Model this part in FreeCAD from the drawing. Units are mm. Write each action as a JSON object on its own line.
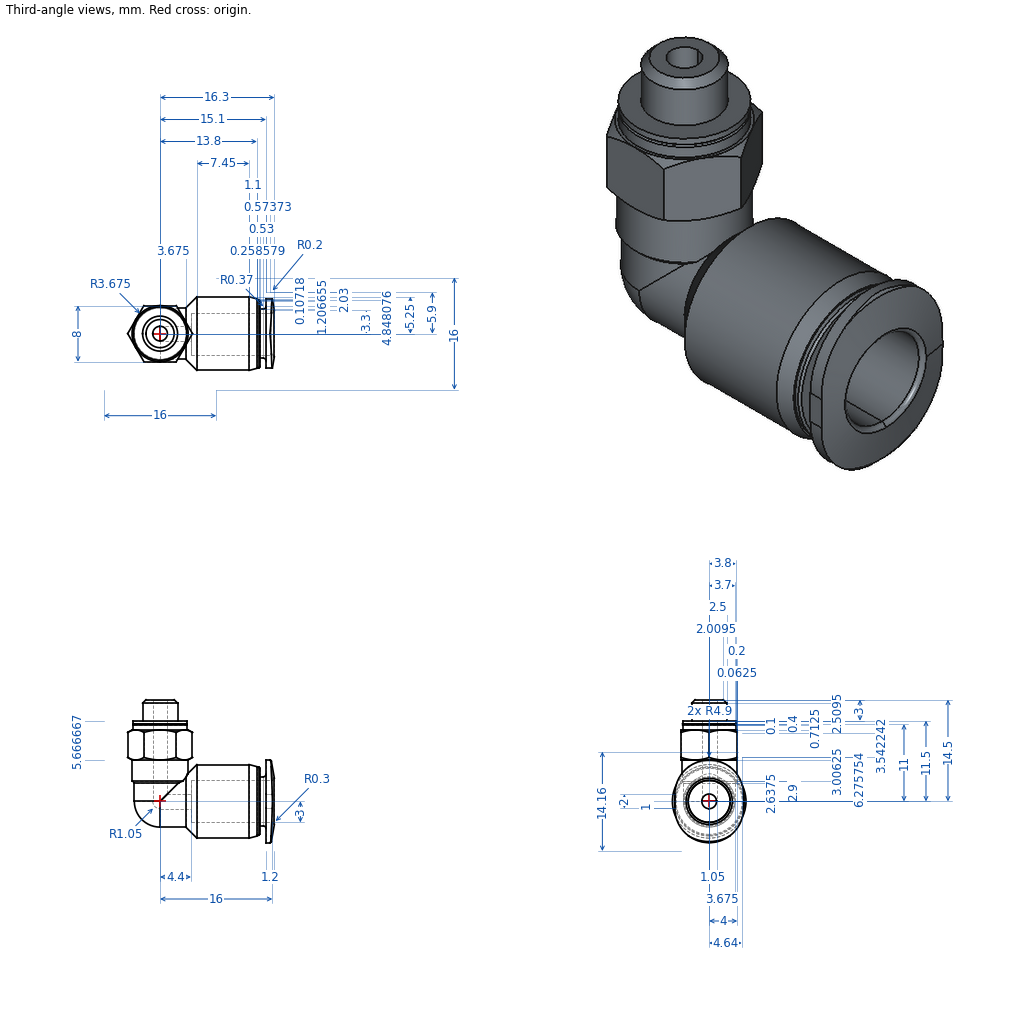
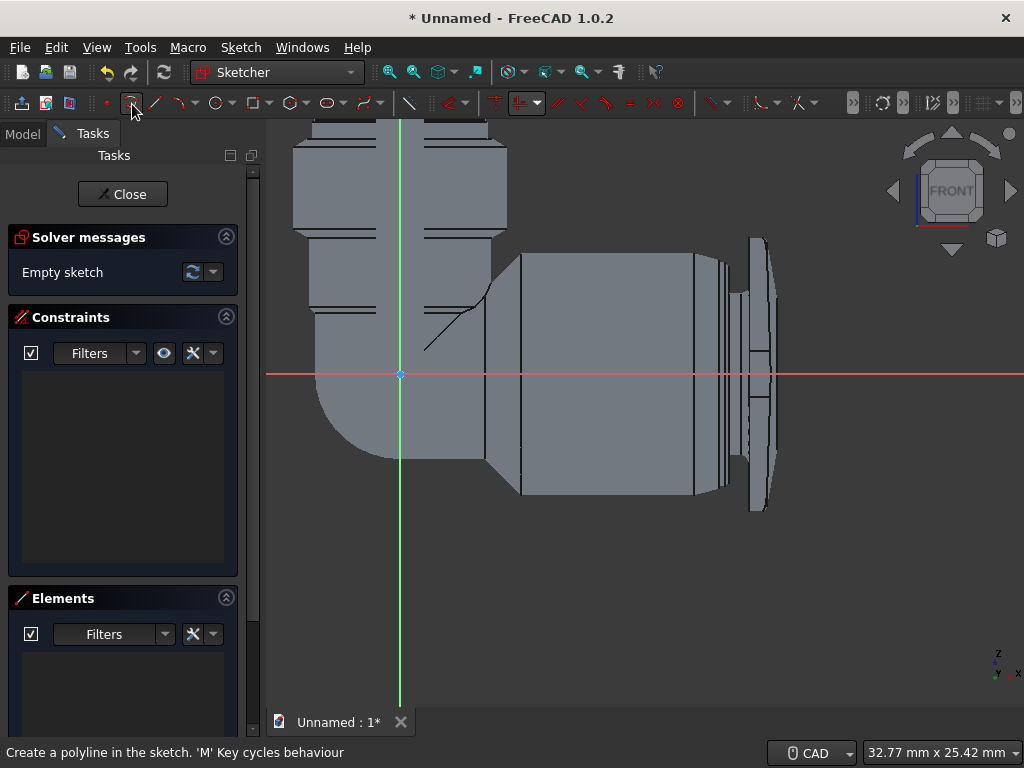
{"action": "left_click", "coordinate": [376, 374]}
{"action": "left_click", "coordinate": [777, 383]}
{"action": "left_click", "coordinate": [777, 451]}
{"action": "right_click", "coordinate": [777, 451]}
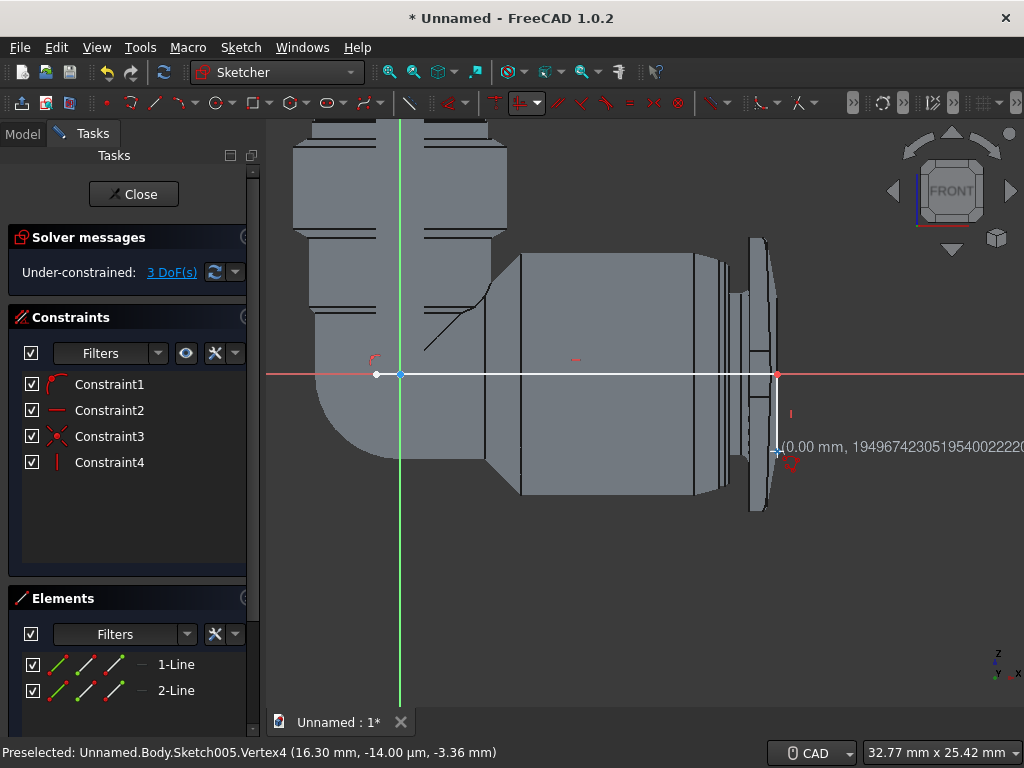
{"action": "scroll", "coordinate": [770, 444], "scroll_direction": "up", "scroll_amount": 5}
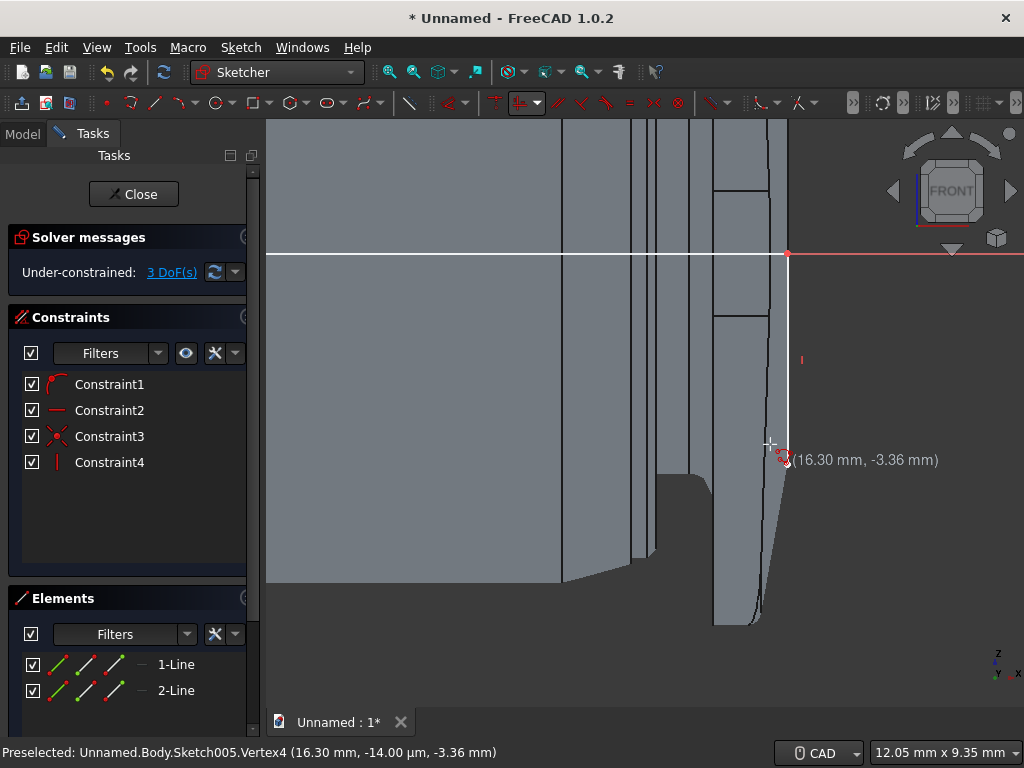
{"action": "left_click", "coordinate": [769, 442]}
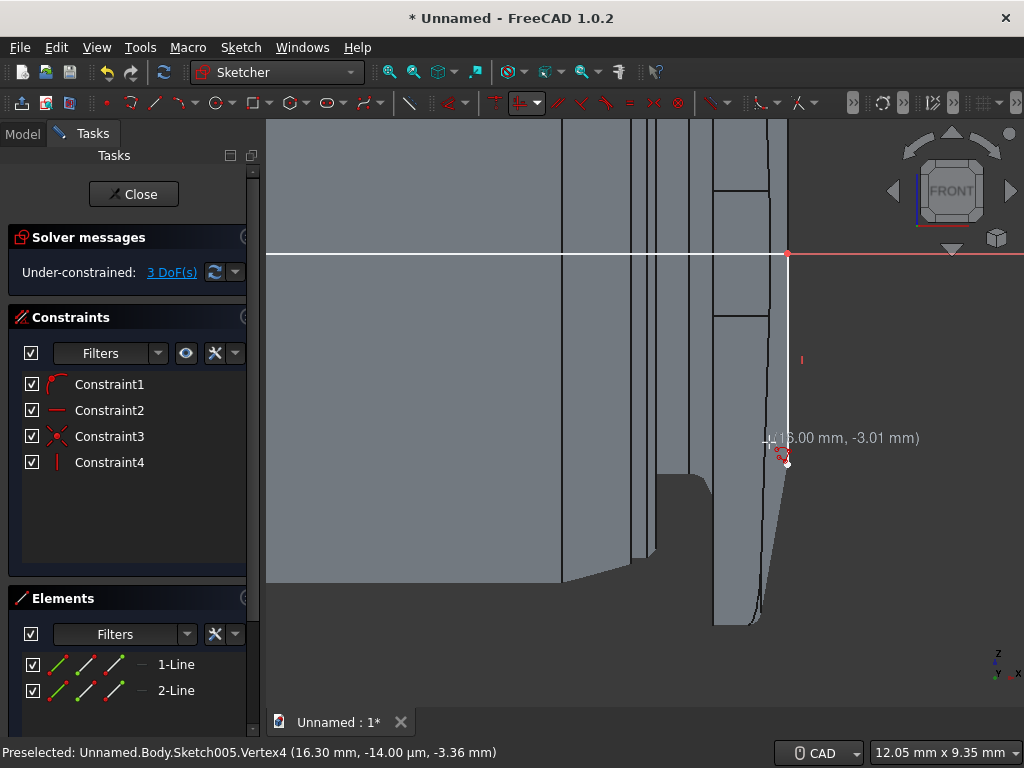
{"action": "scroll", "coordinate": [771, 445], "scroll_direction": "down", "scroll_amount": 5}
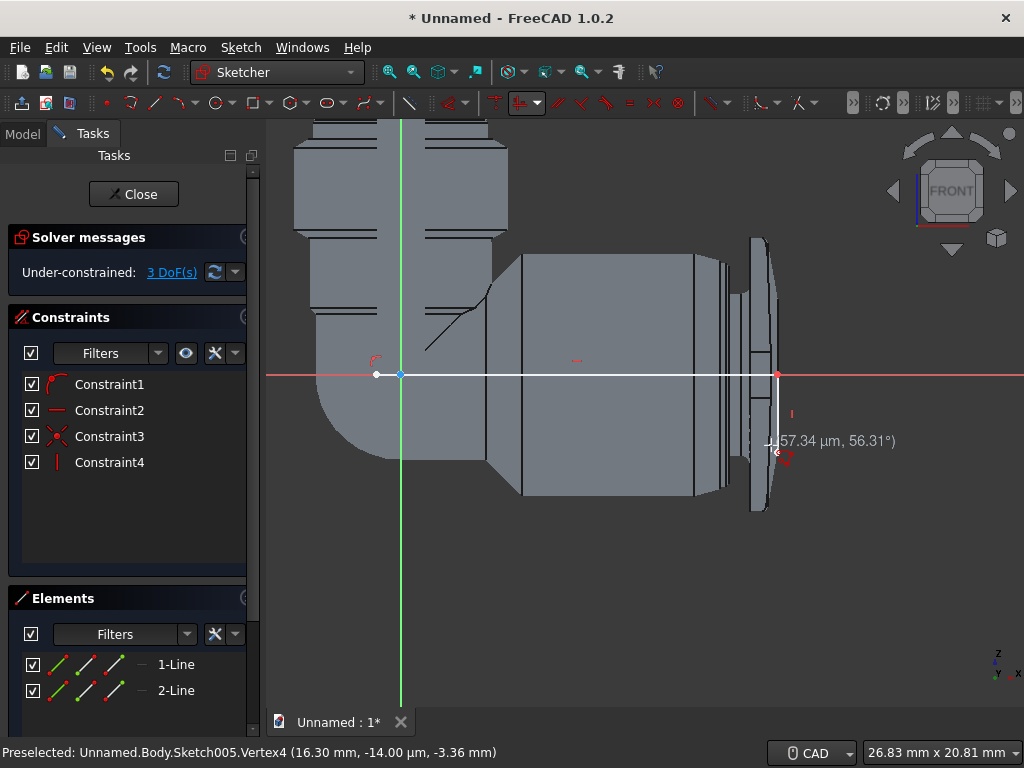
{"action": "left_click", "coordinate": [502, 444]}
{"action": "left_click", "coordinate": [502, 399]}
{"action": "left_click", "coordinate": [401, 399]}
{"action": "right_click", "coordinate": [401, 399]}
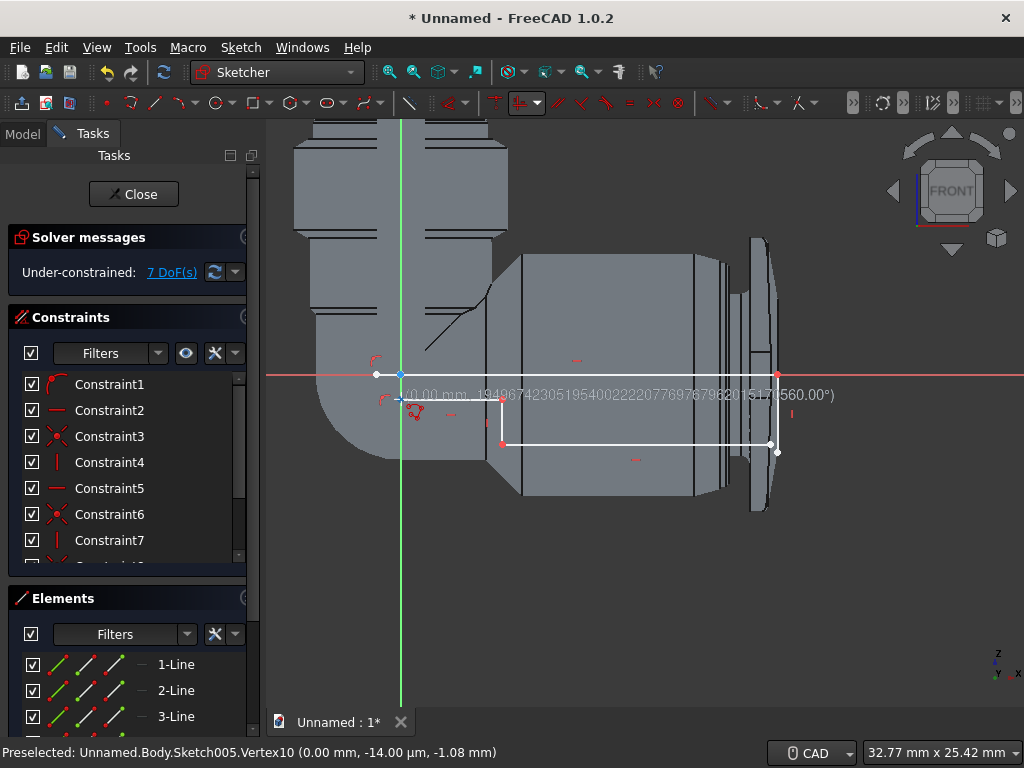
{"action": "left_click", "coordinate": [180, 104]}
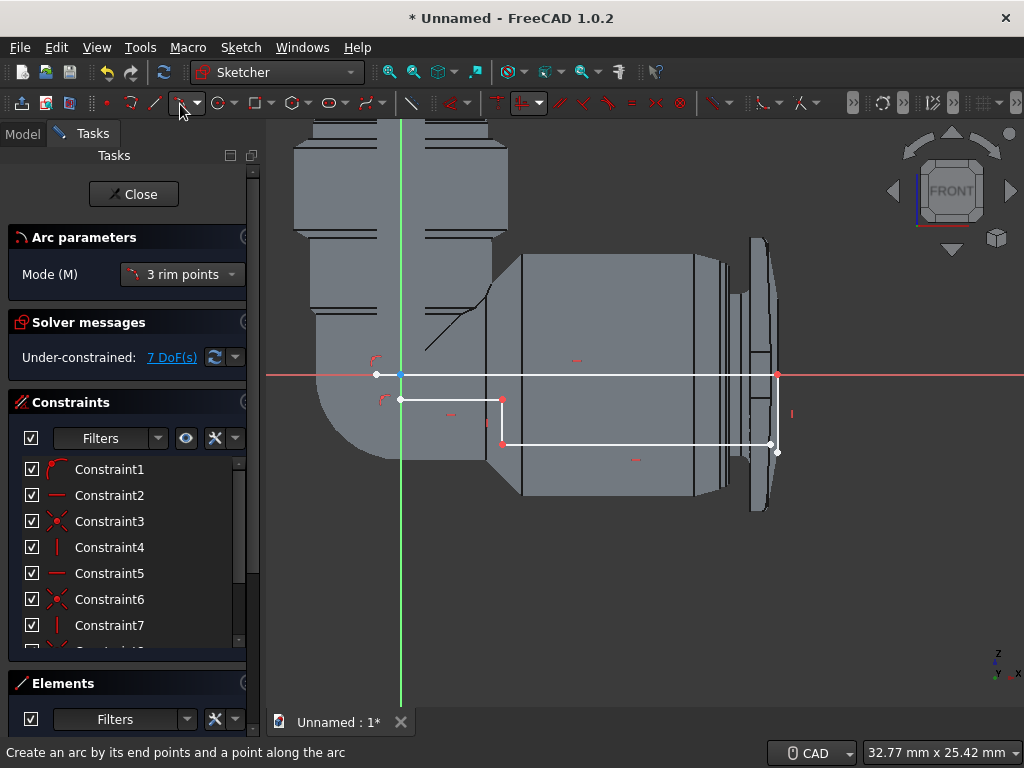
{"action": "scroll", "coordinate": [778, 451], "scroll_direction": "up", "scroll_amount": 3}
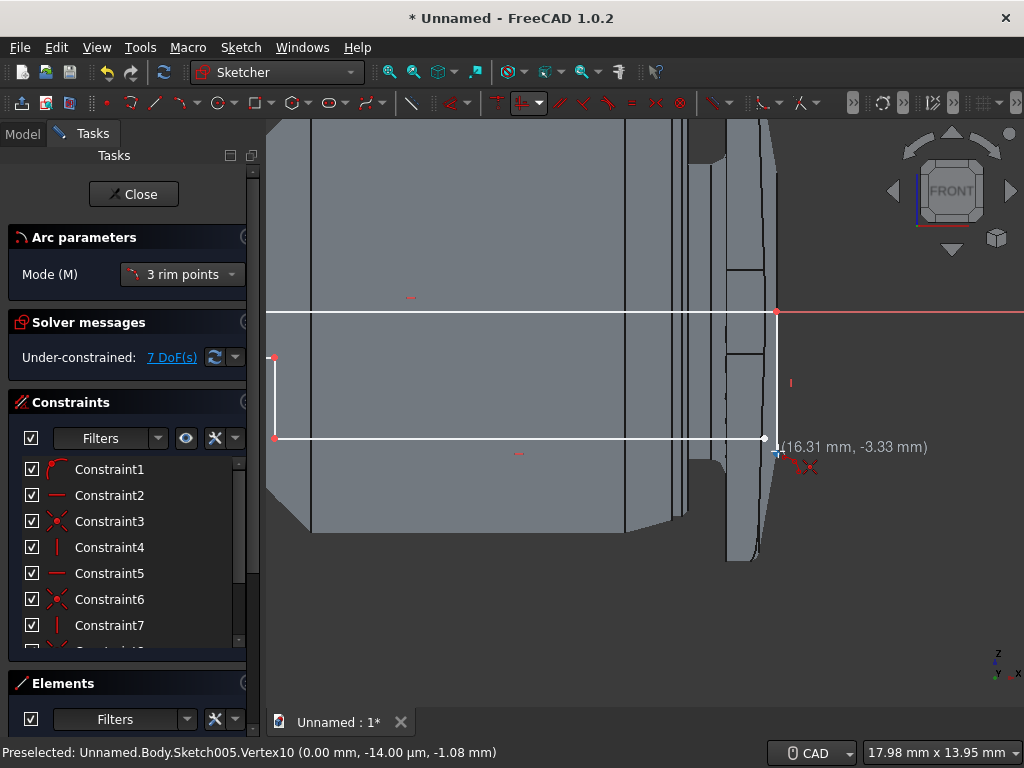
{"action": "left_click", "coordinate": [777, 454]}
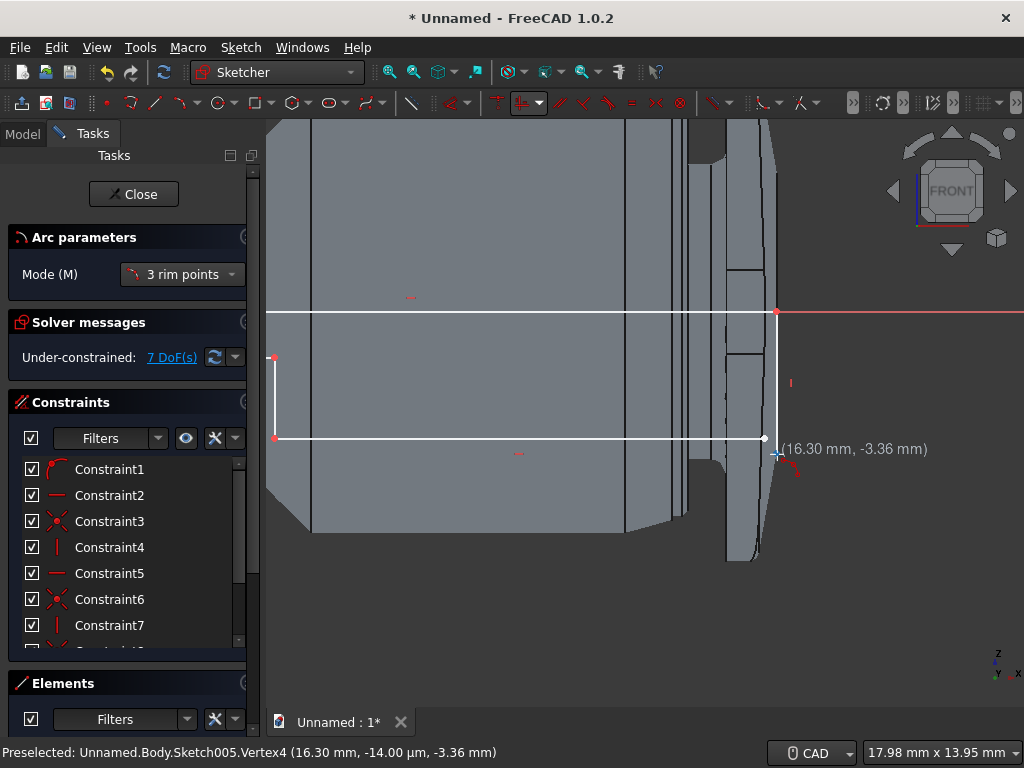
{"action": "scroll", "coordinate": [764, 438], "scroll_direction": "up", "scroll_amount": 2}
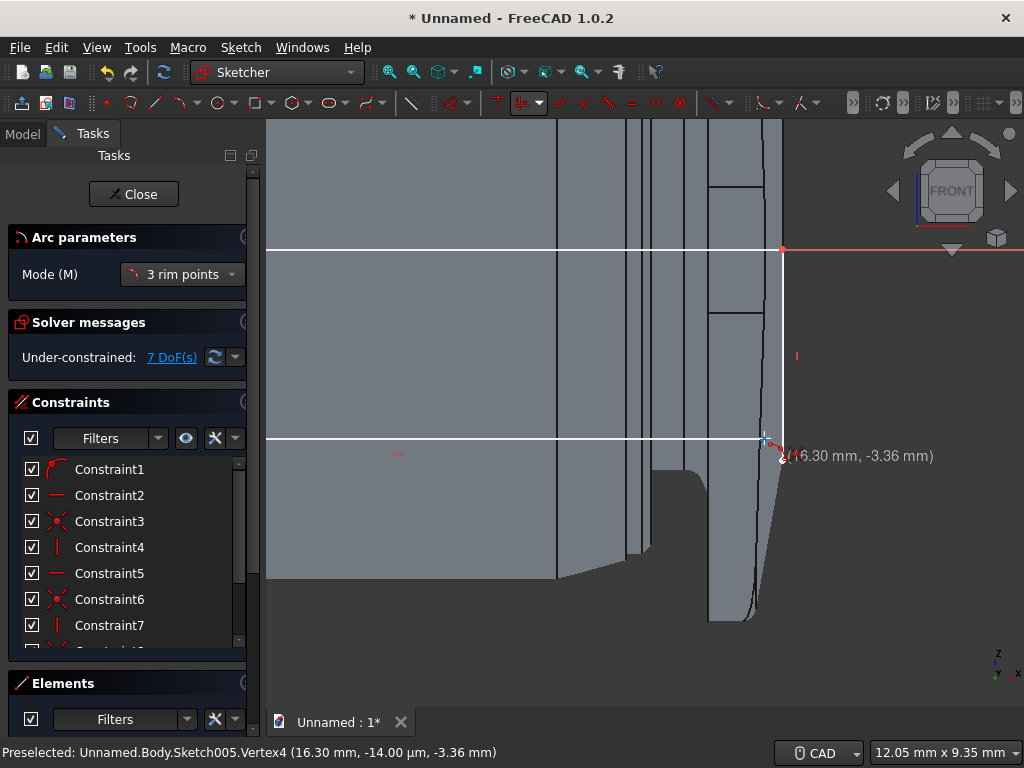
{"action": "left_click", "coordinate": [764, 439]}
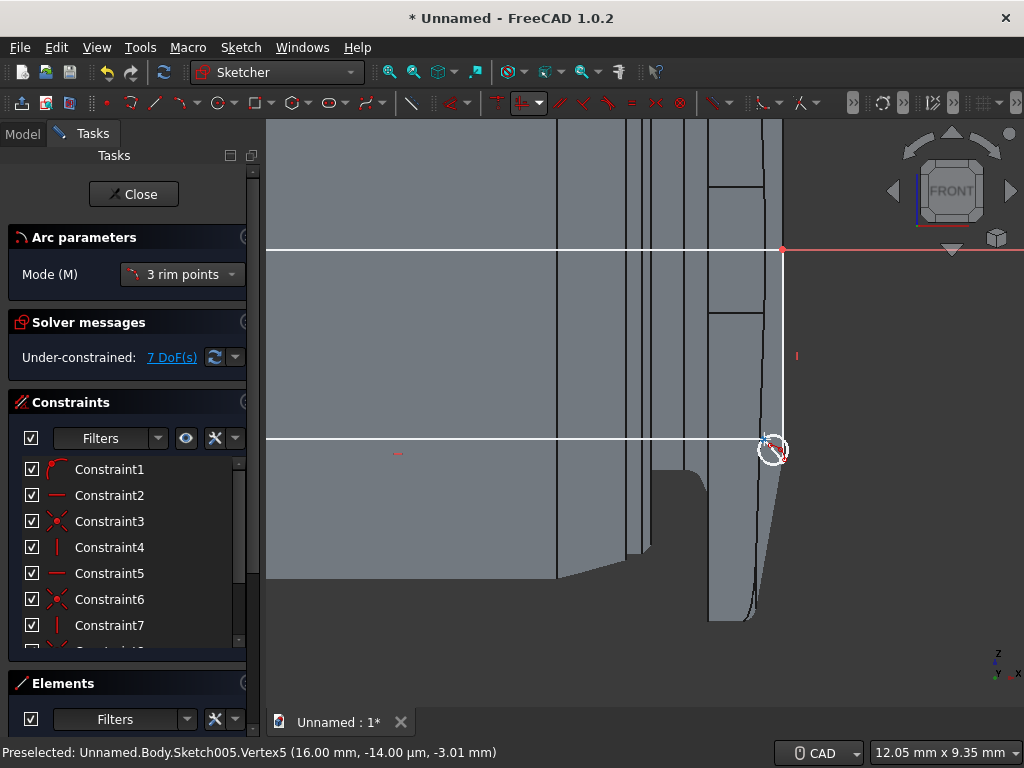
{"action": "scroll", "coordinate": [777, 444], "scroll_direction": "up", "scroll_amount": 6}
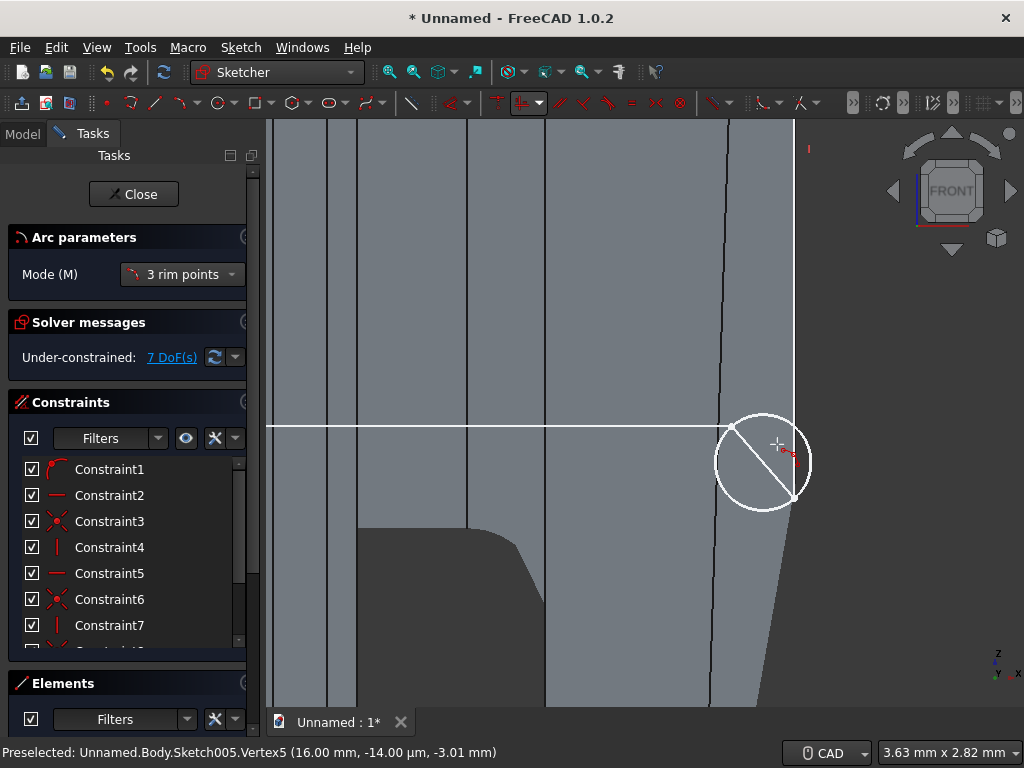
{"action": "left_click", "coordinate": [777, 442]}